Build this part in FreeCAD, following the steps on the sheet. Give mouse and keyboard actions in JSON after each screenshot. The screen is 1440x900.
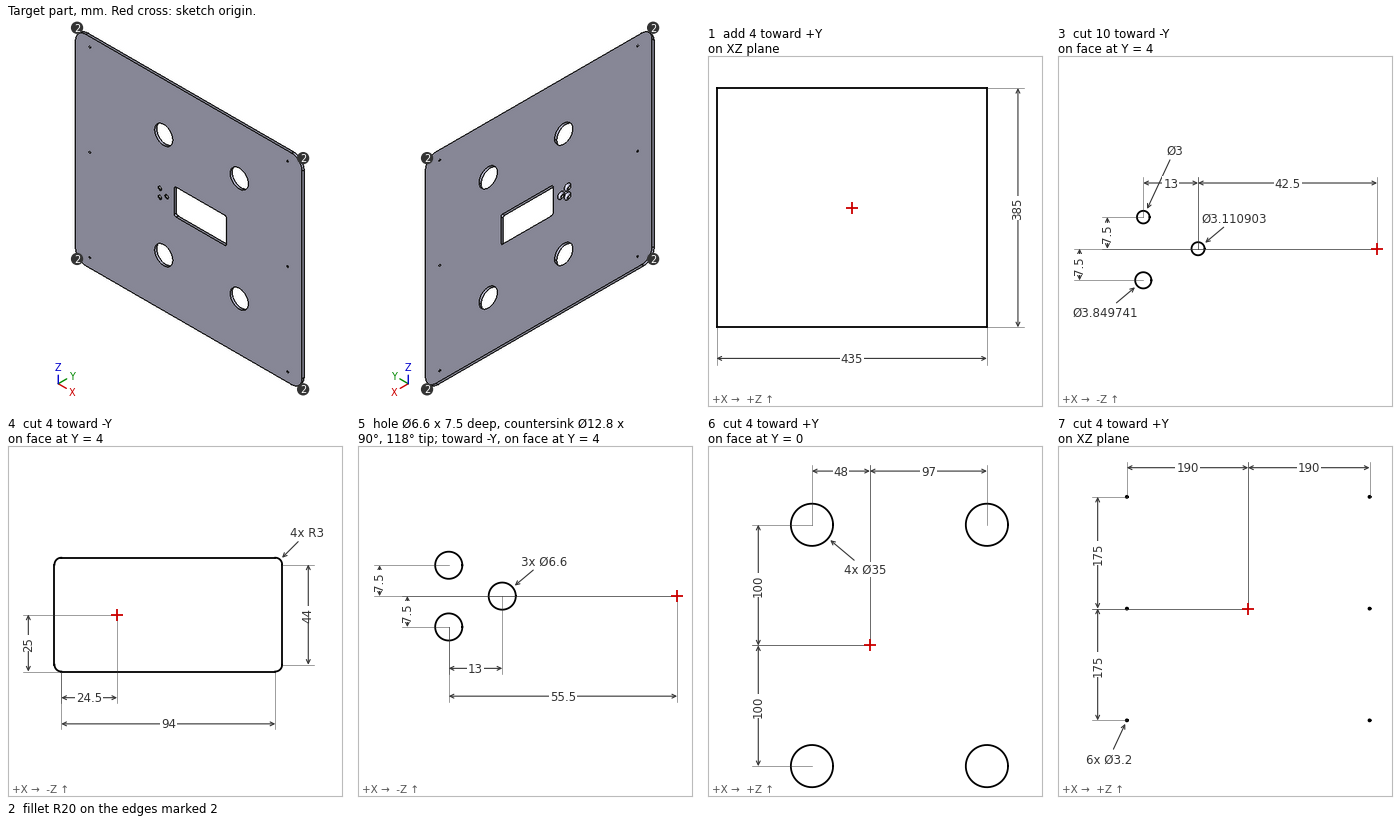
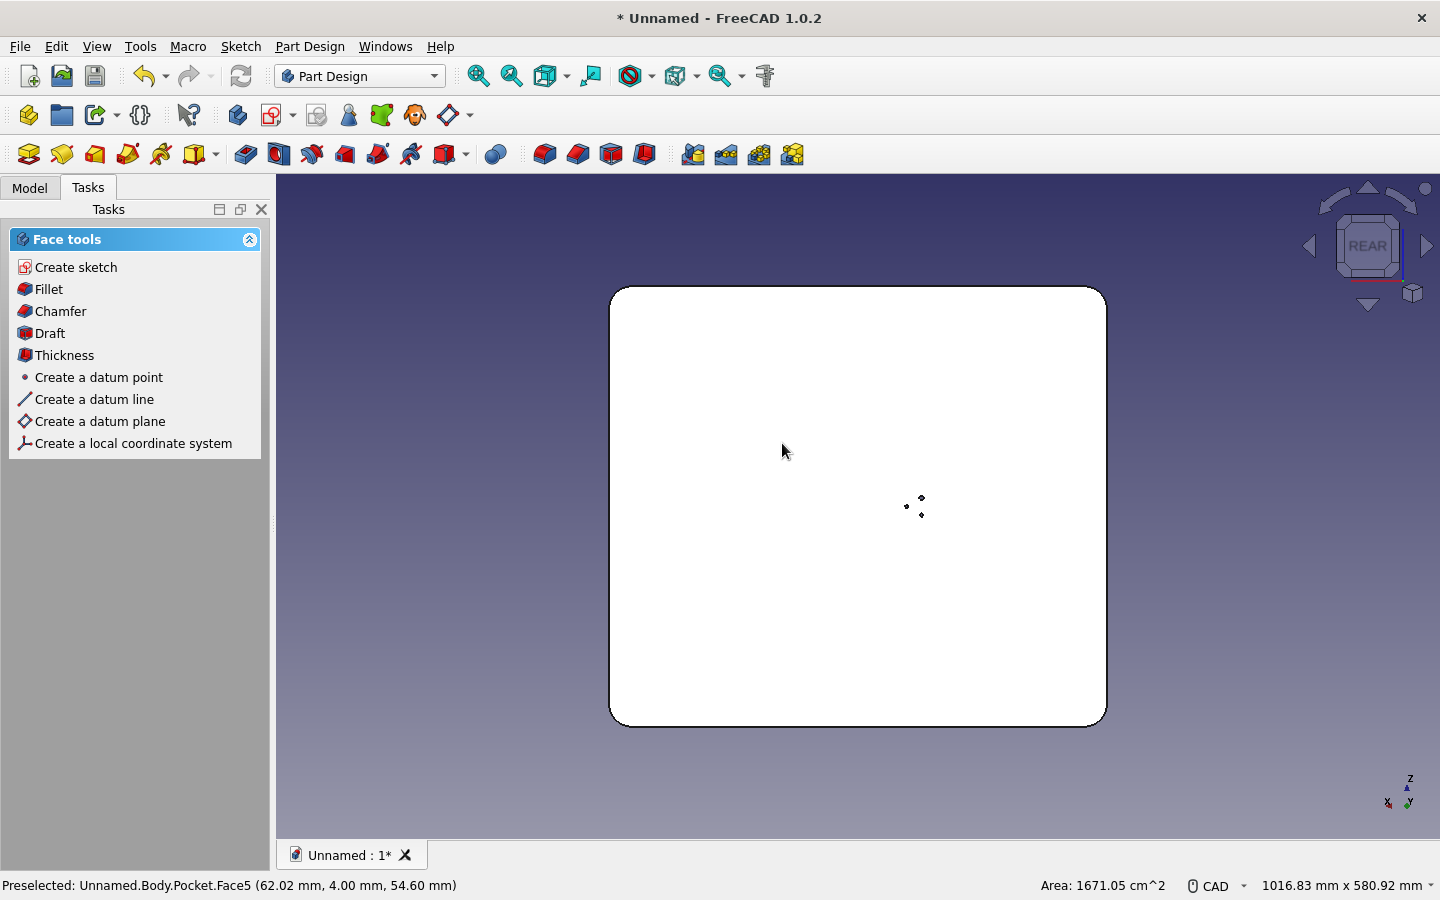
{"action": "left_click", "coordinate": [270, 116]}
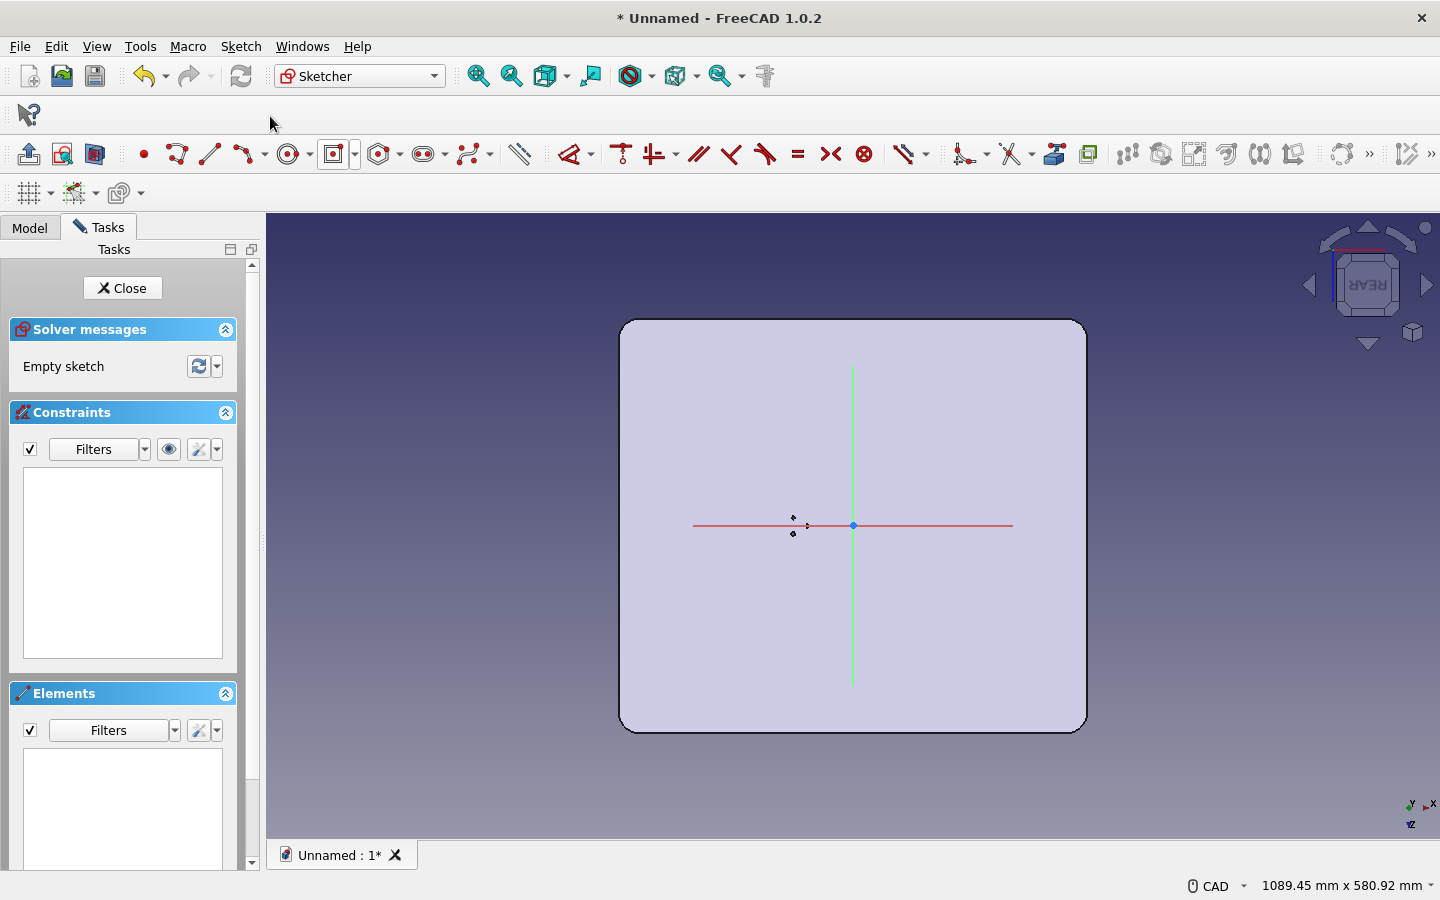
{"action": "scroll", "coordinate": [896, 526], "scroll_direction": "up", "scroll_amount": 9}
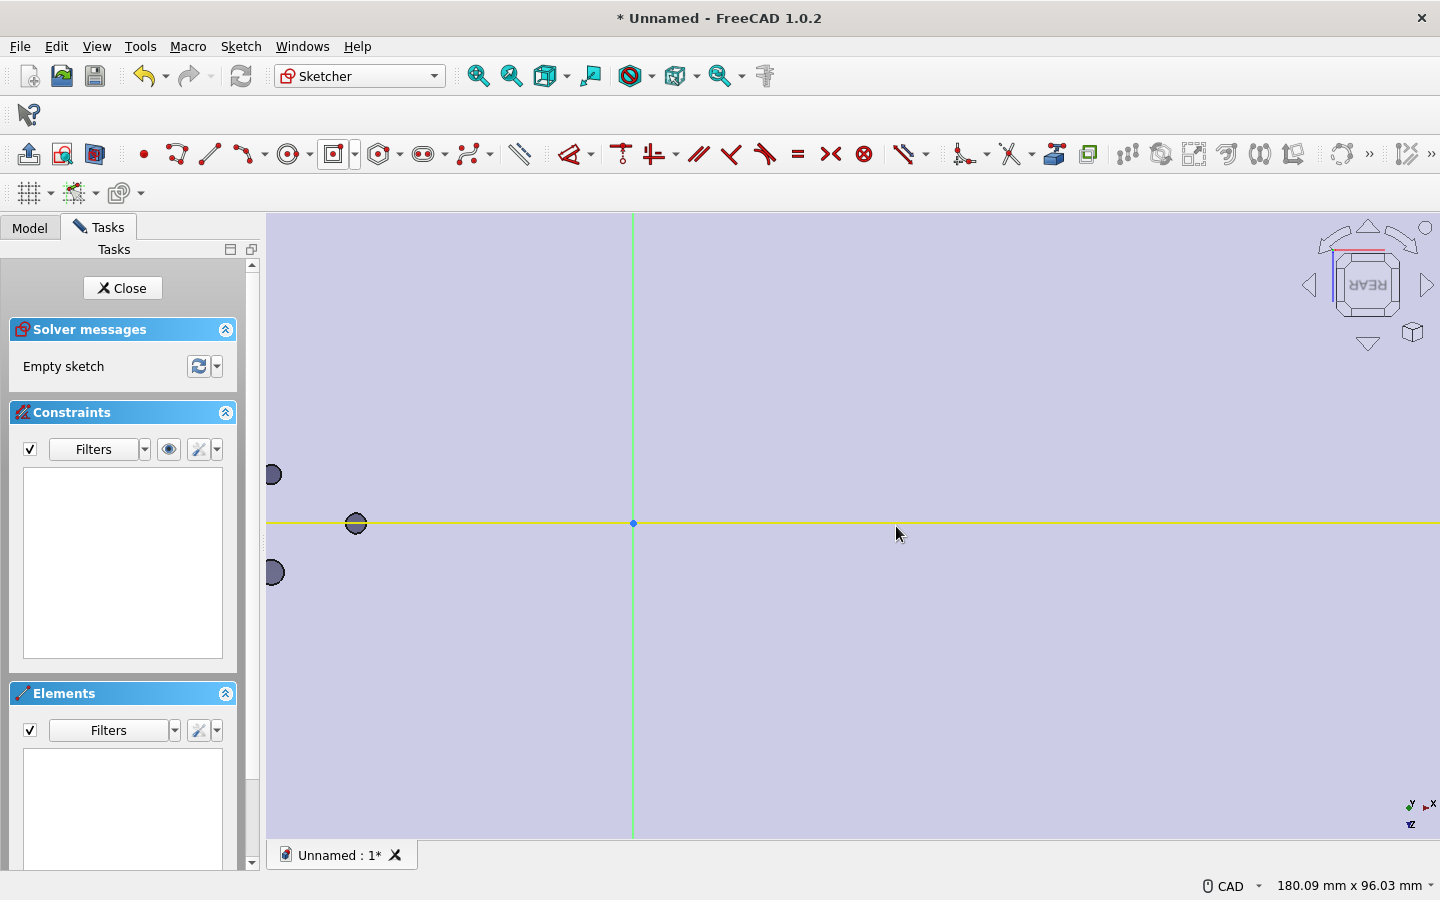
{"action": "left_click", "coordinate": [210, 154]}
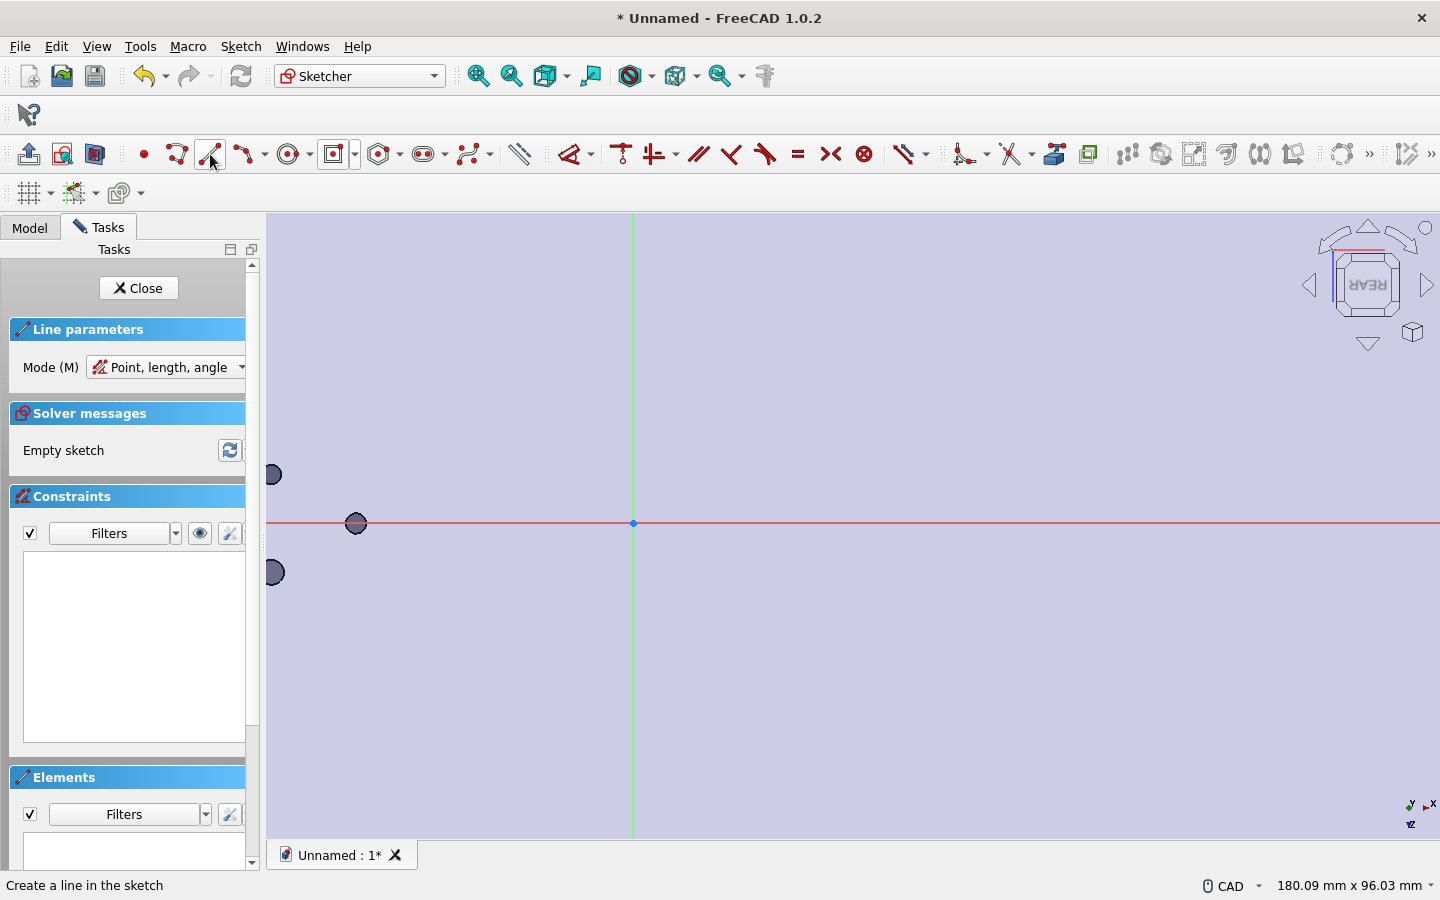
{"action": "left_click", "coordinate": [473, 686]}
{"action": "left_click", "coordinate": [1086, 686]}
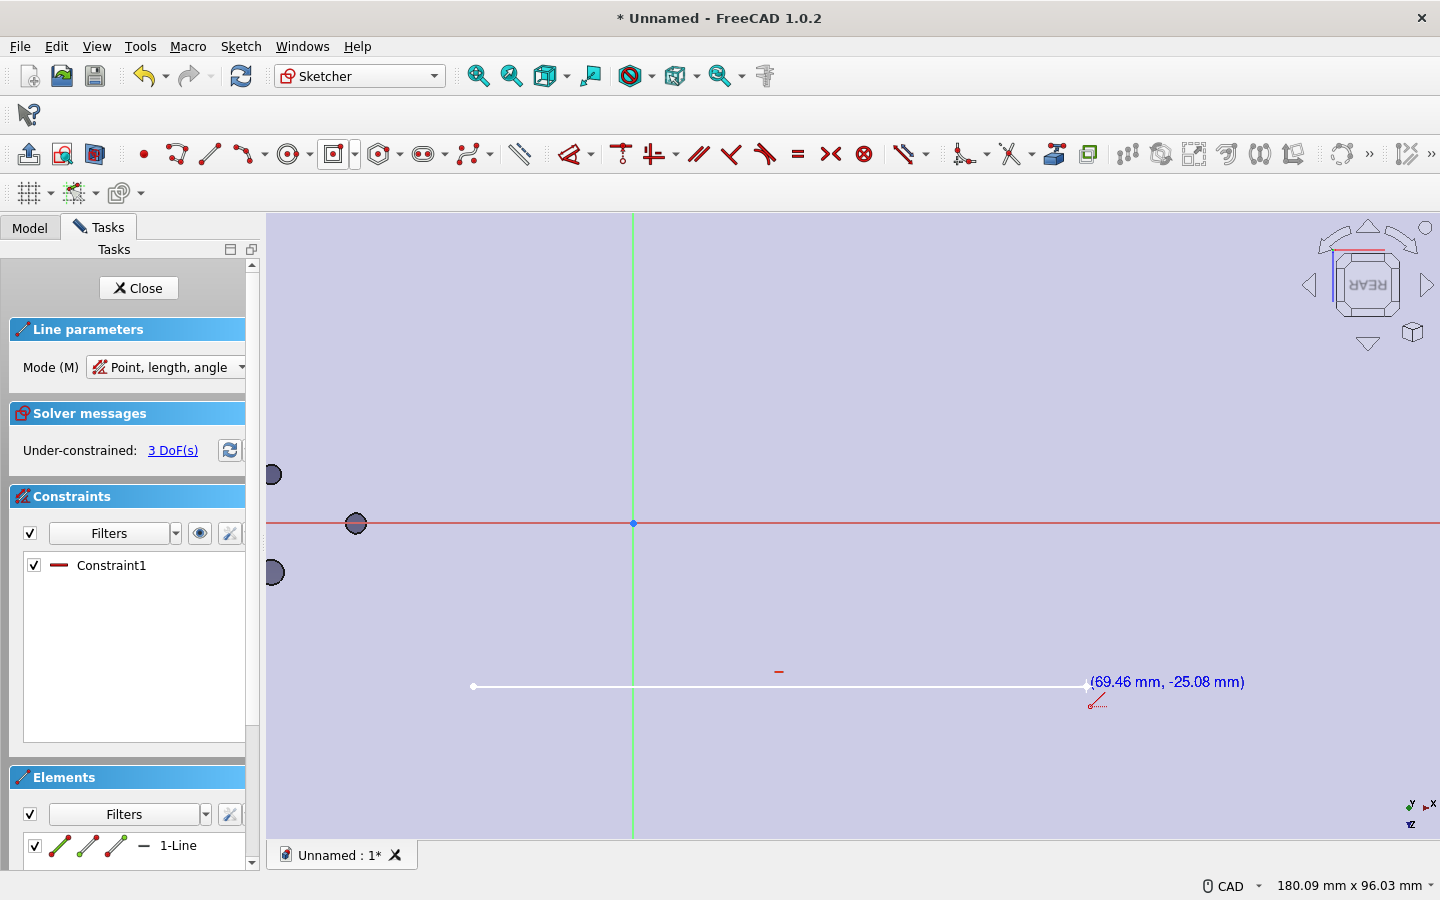
{"action": "left_click", "coordinate": [1106, 667]}
{"action": "left_click", "coordinate": [1106, 380]}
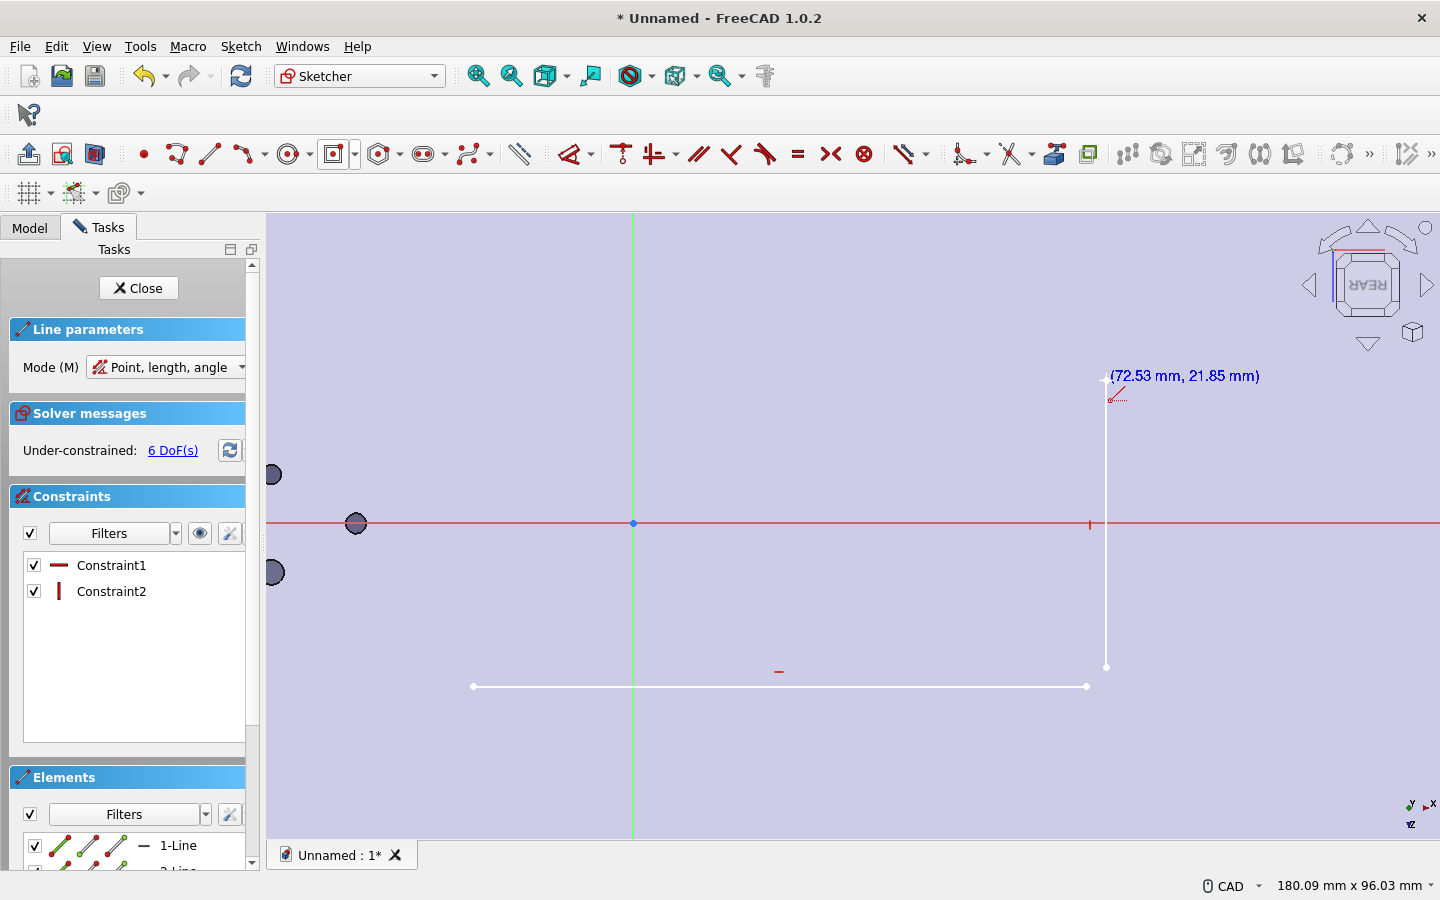
{"action": "left_click", "coordinate": [1086, 360]}
{"action": "left_click", "coordinate": [473, 360]}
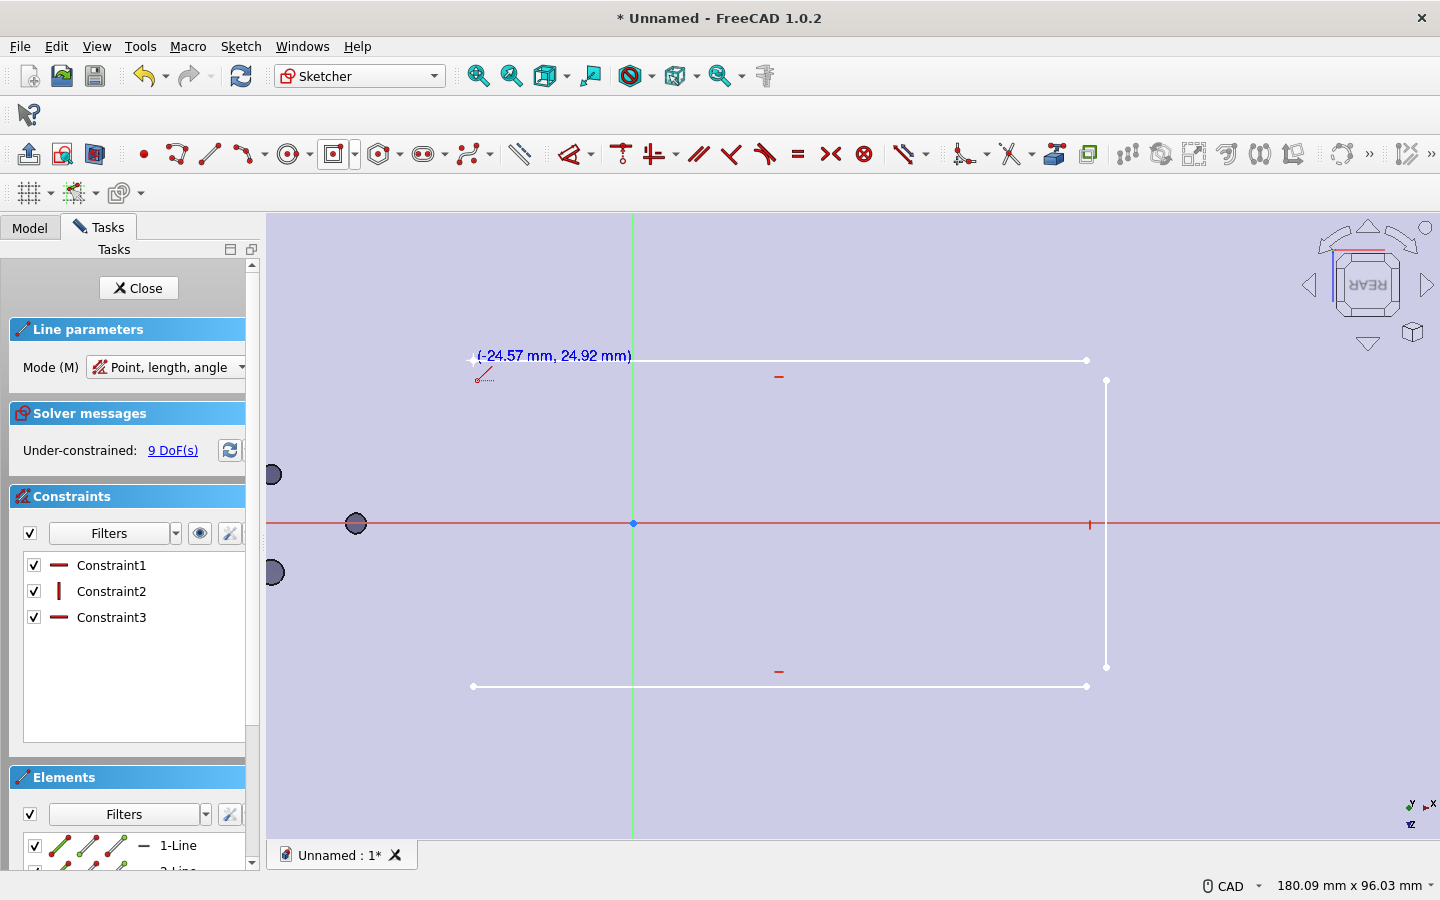
{"action": "left_click", "coordinate": [454, 380]}
{"action": "left_click", "coordinate": [454, 667]}